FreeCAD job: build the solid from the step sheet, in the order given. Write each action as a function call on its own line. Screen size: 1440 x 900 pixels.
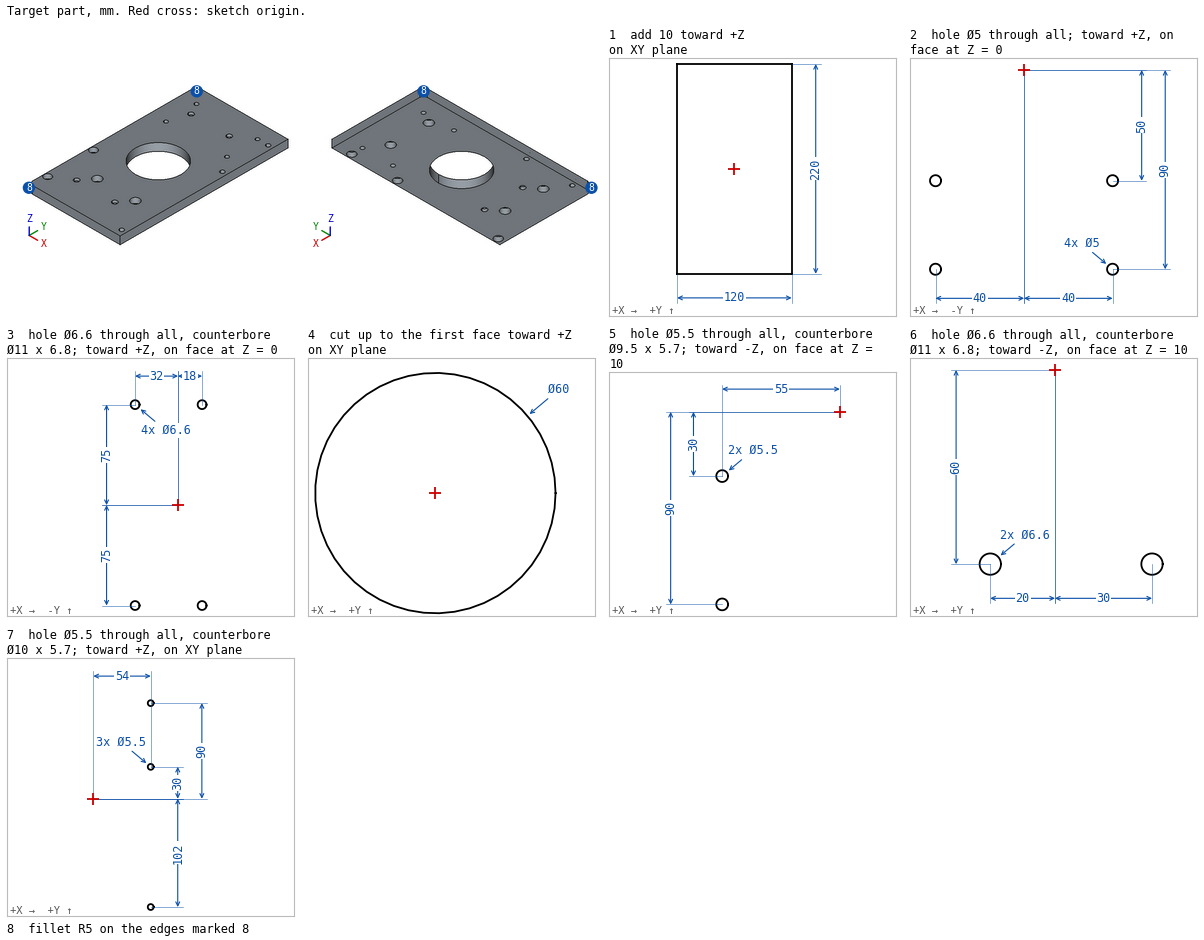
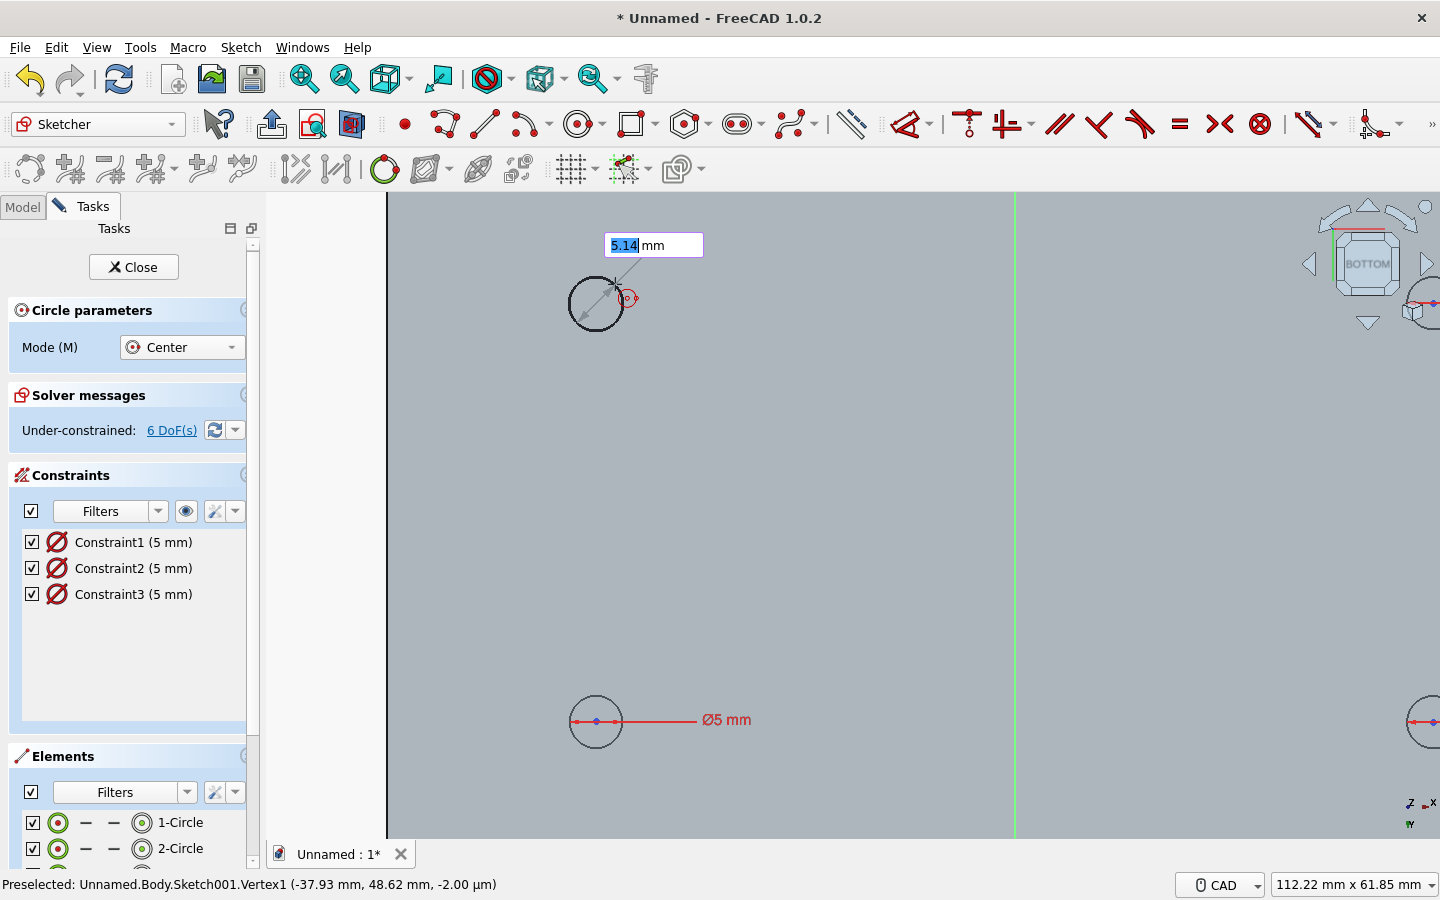
text(5)
key(Return)
key(Escape)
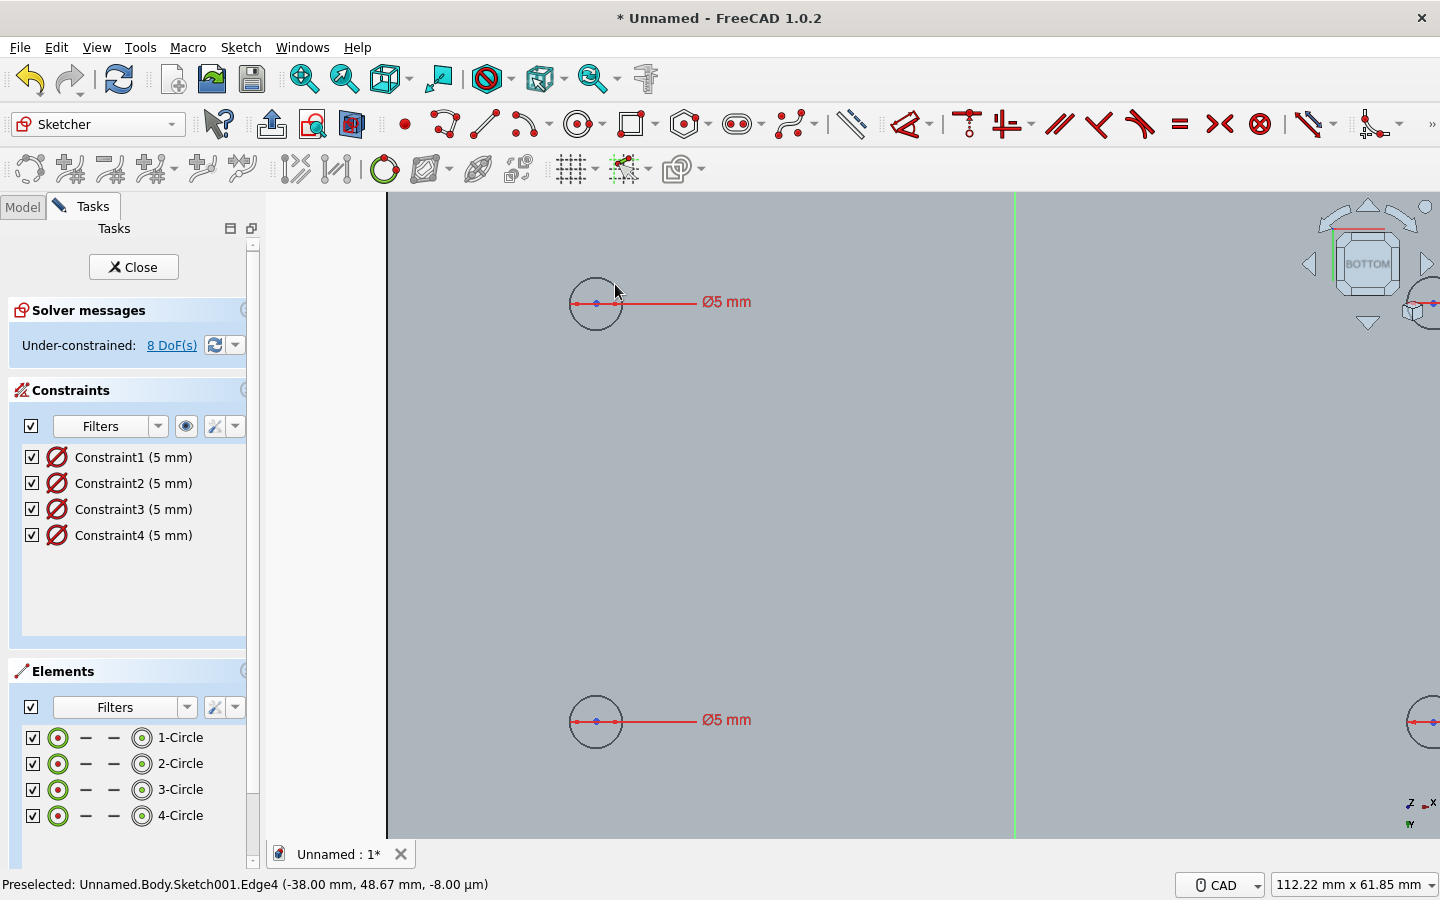
scroll(597, 721, down, 4)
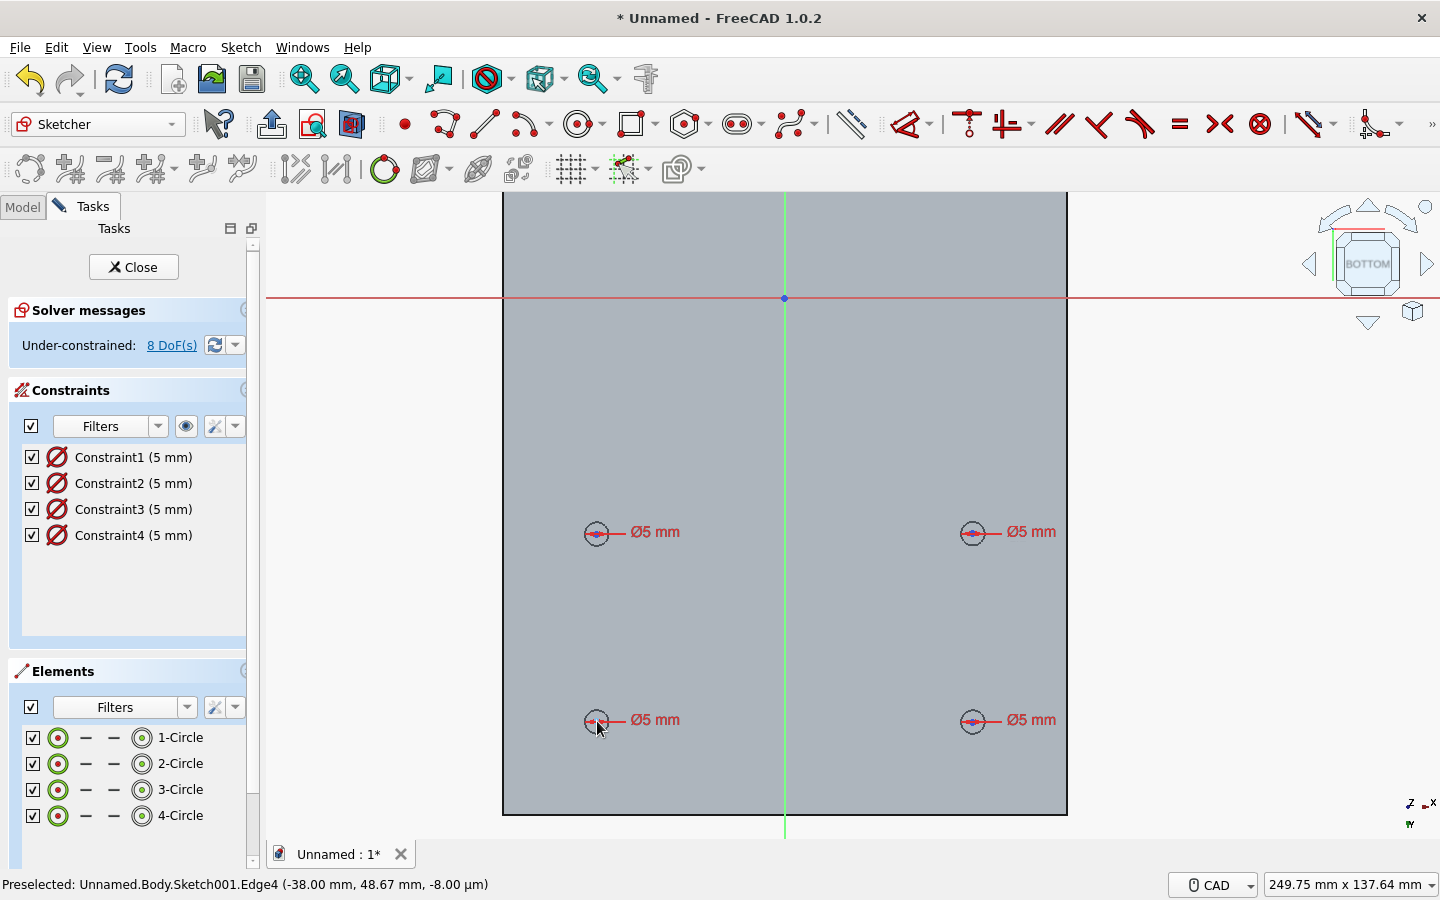
click(973, 722)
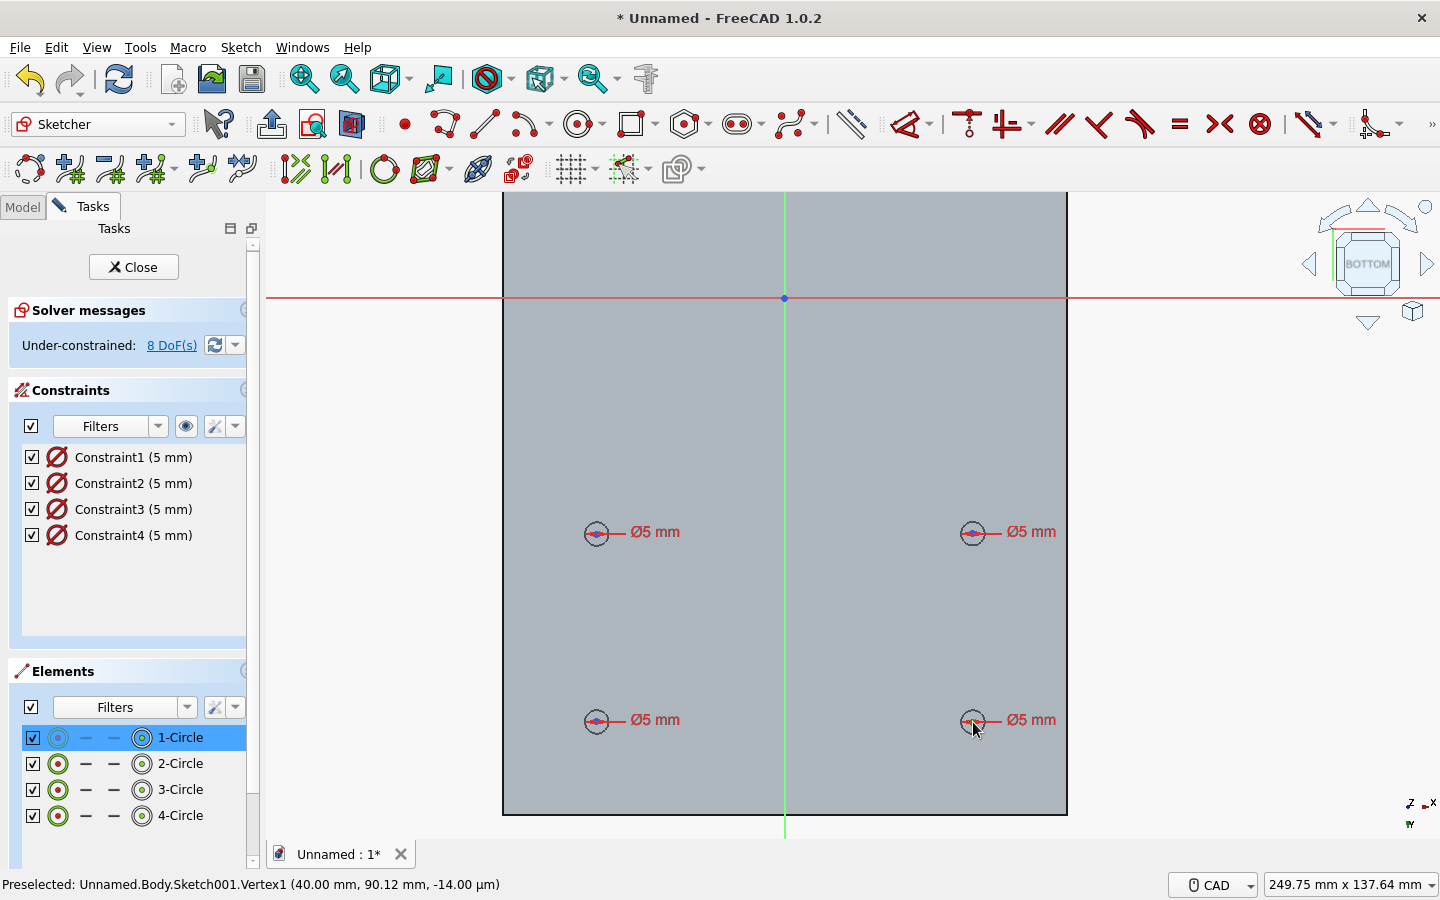
click(973, 534)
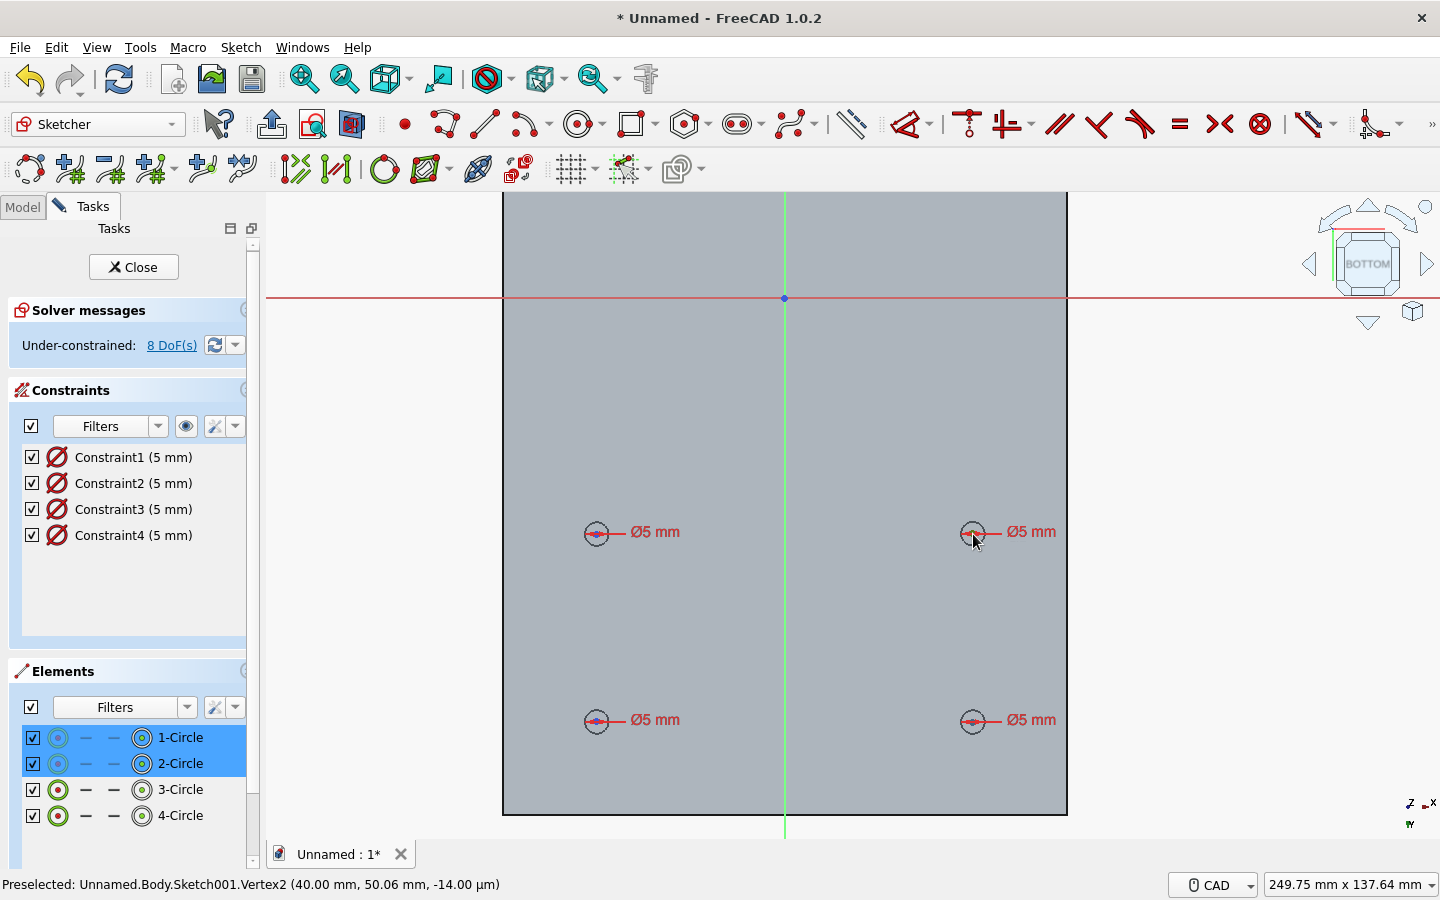
click(1034, 124)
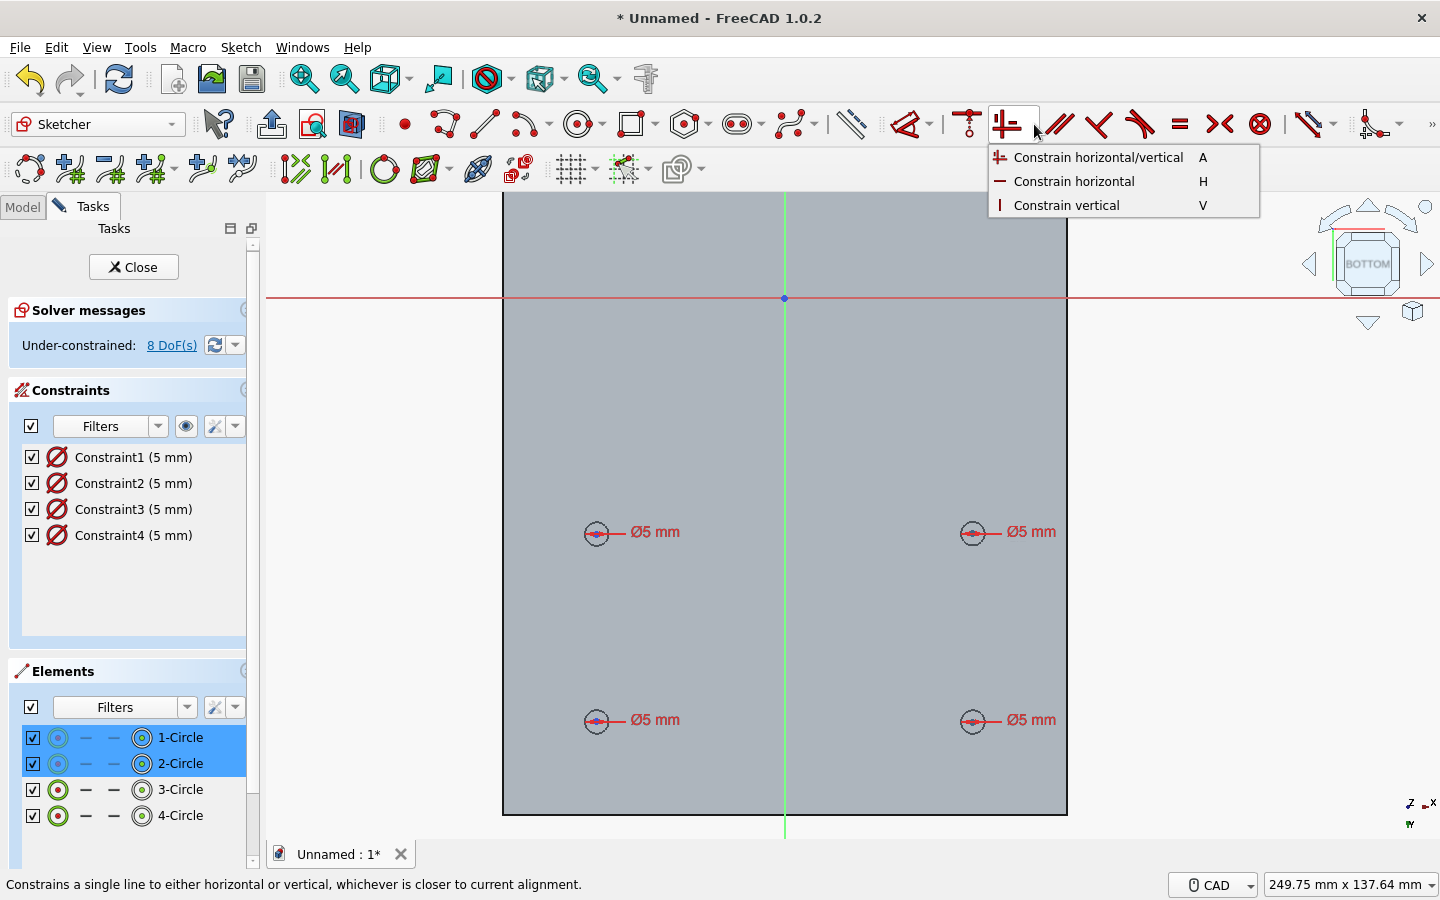
click(1124, 205)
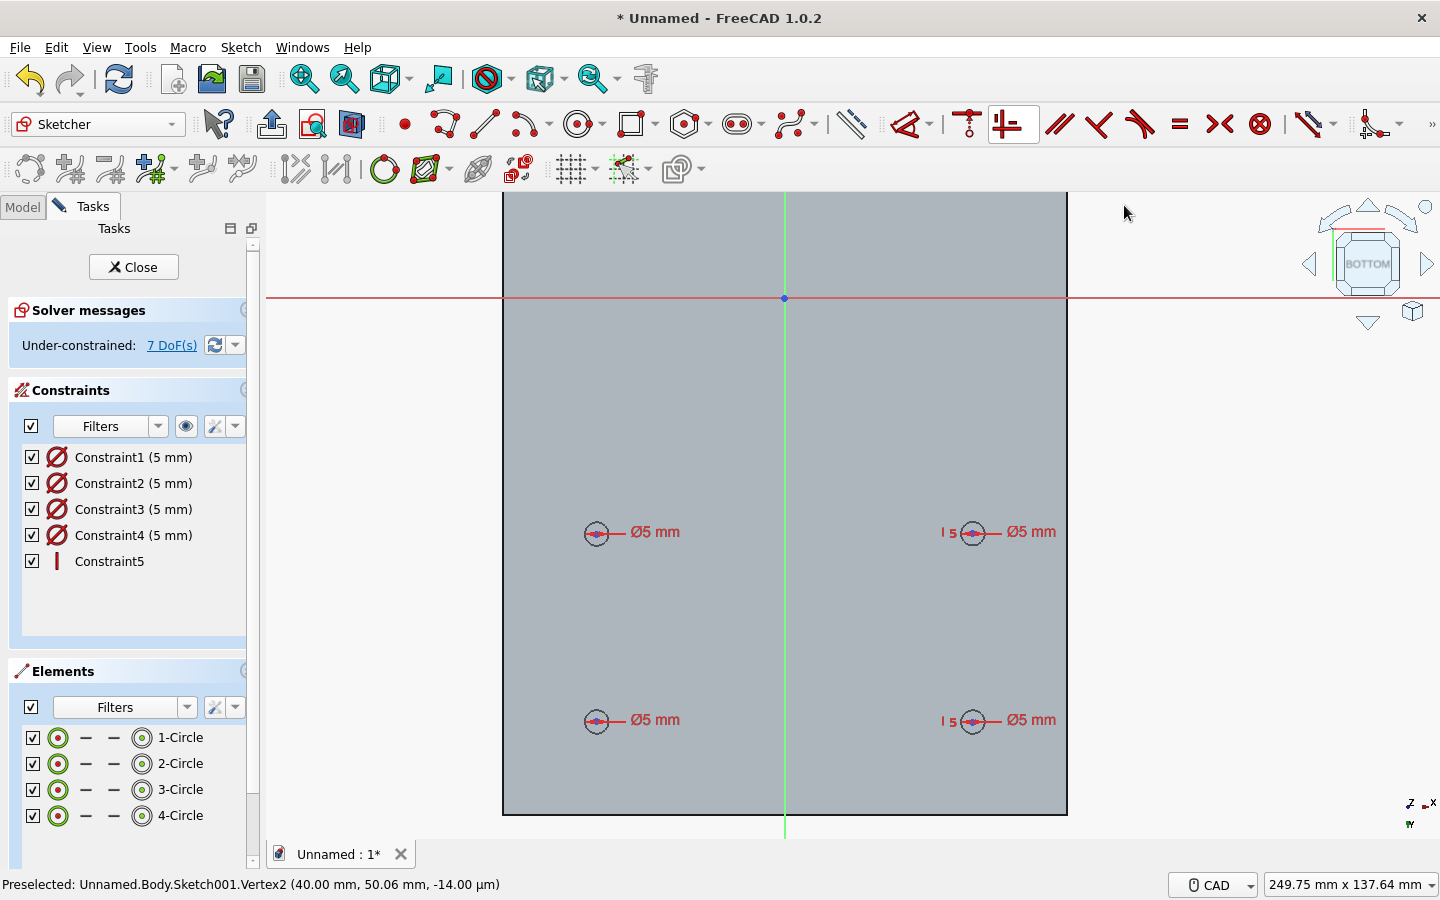
click(973, 722)